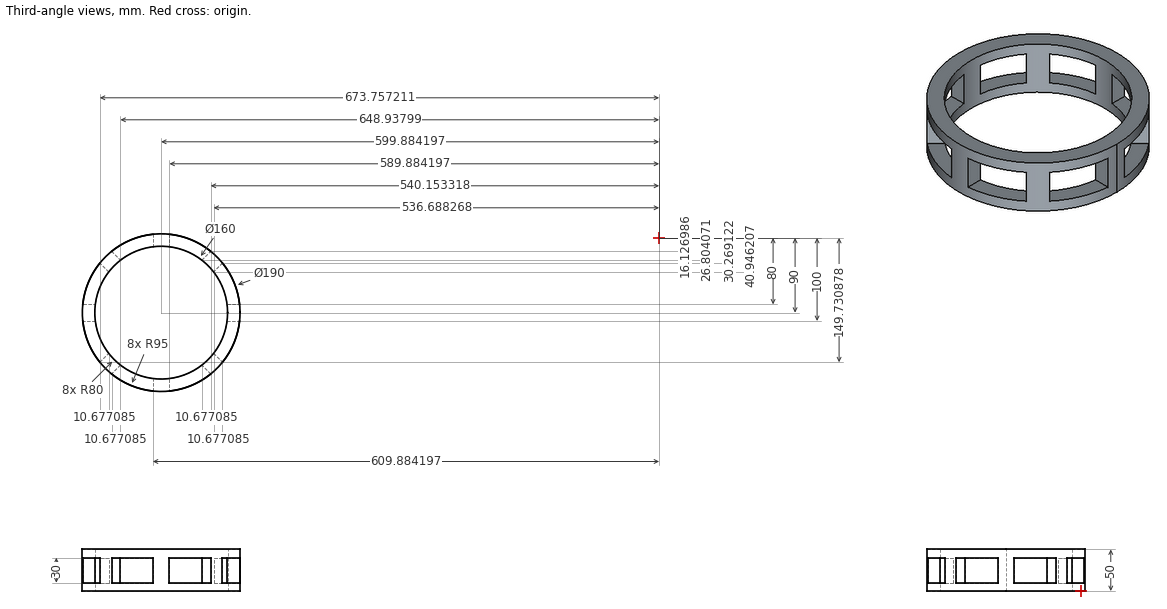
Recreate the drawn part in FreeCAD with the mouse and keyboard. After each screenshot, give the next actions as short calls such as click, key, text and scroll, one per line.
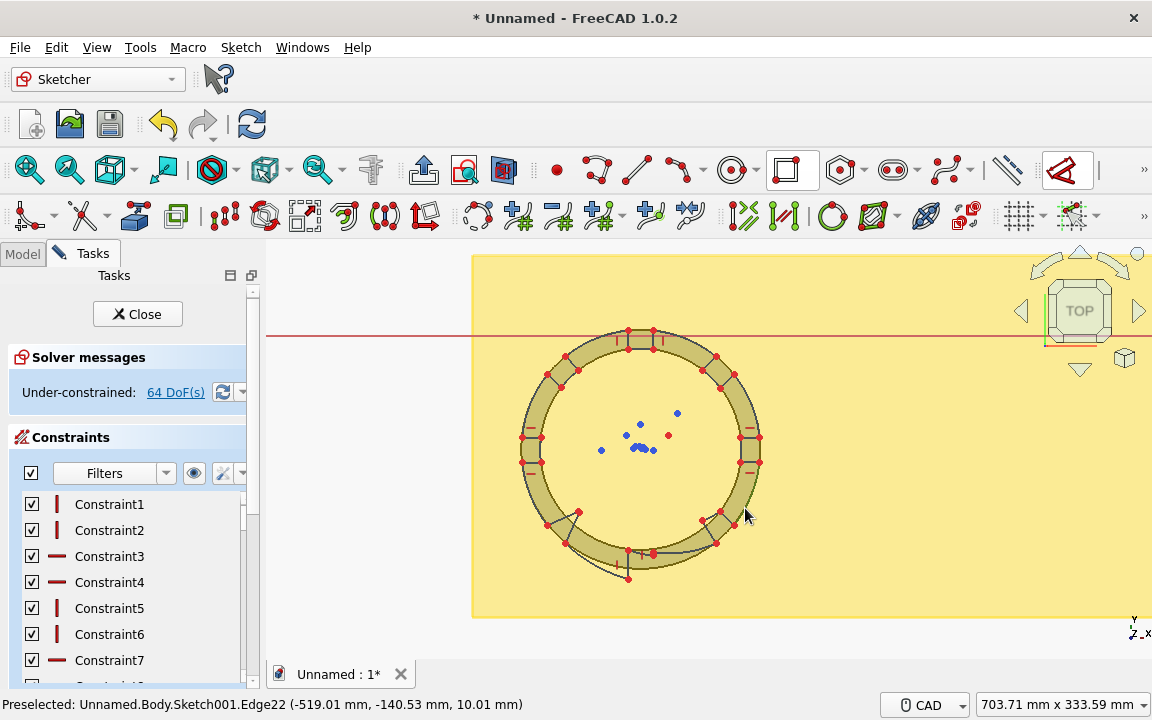
key(c)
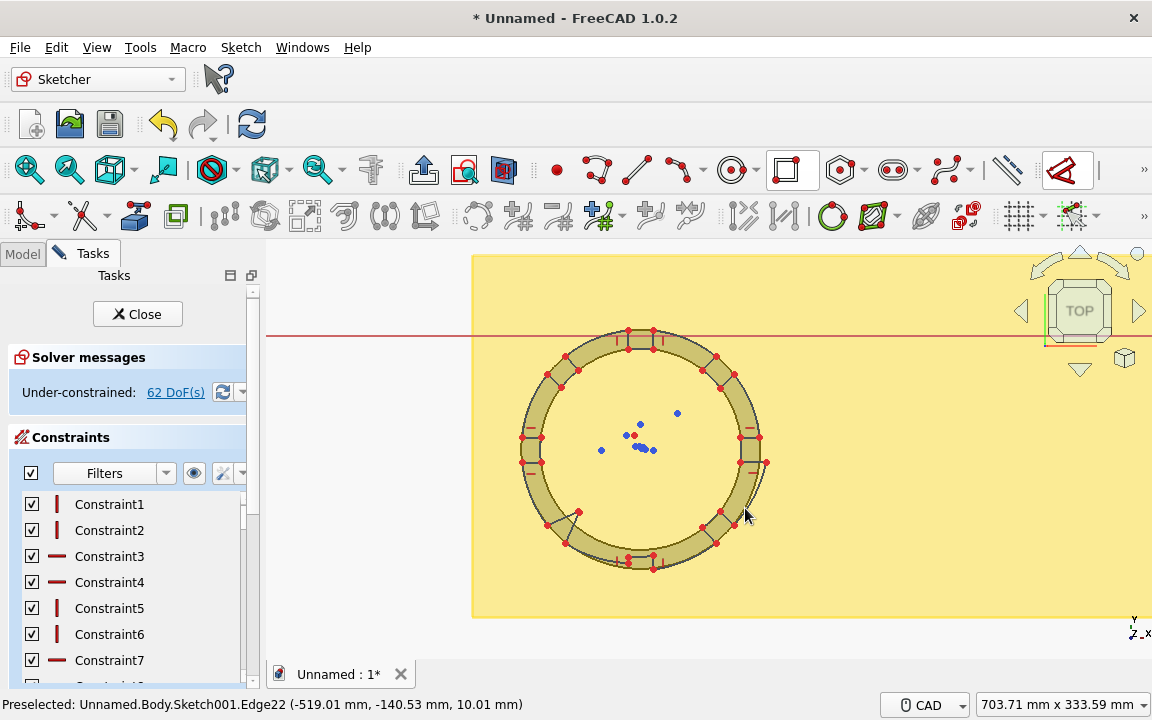
scroll(579, 512, up, 15)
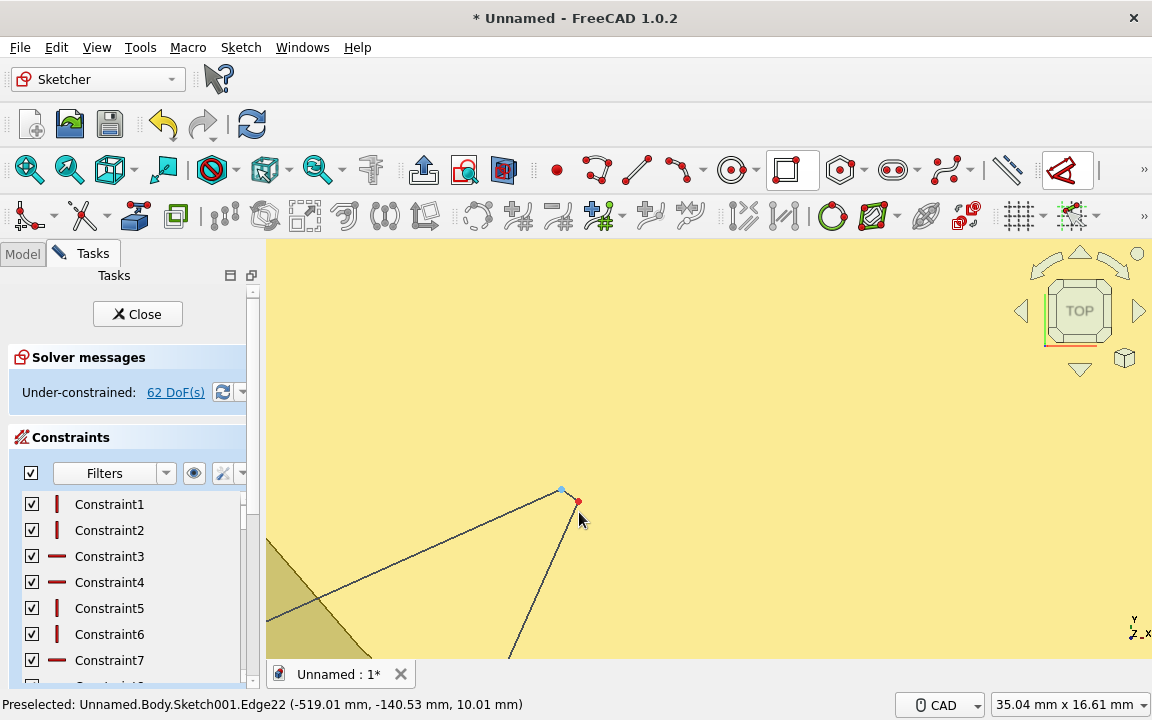
click(570, 495)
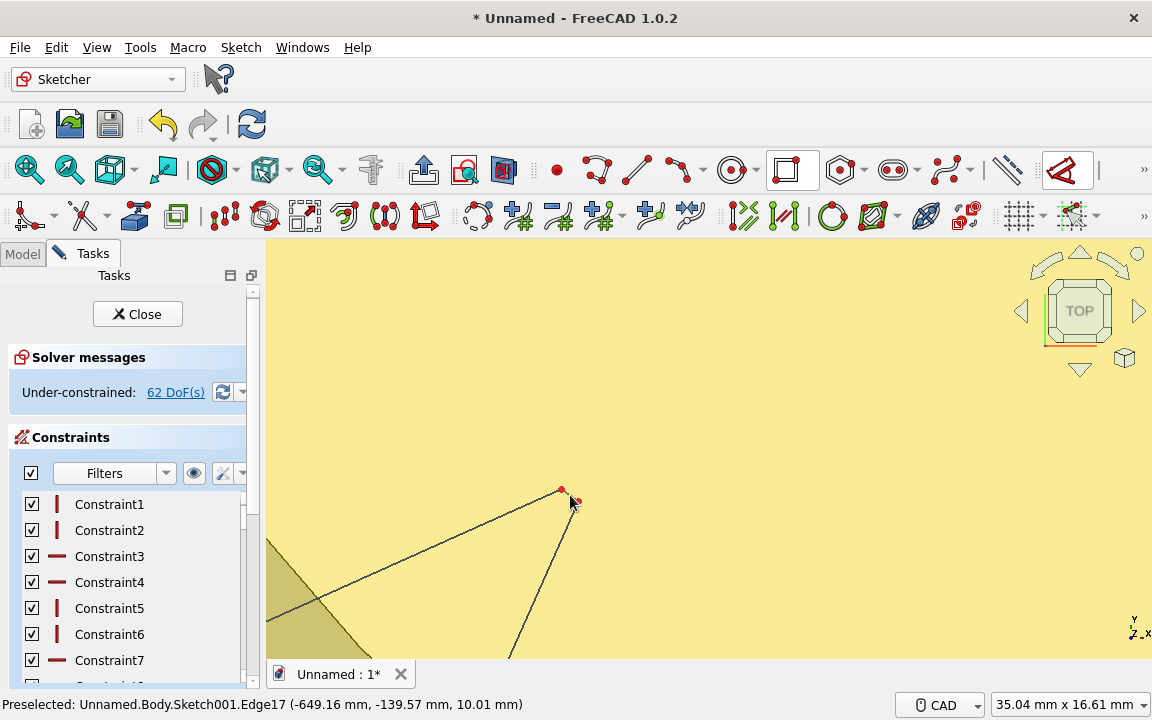
scroll(579, 512, down, 15)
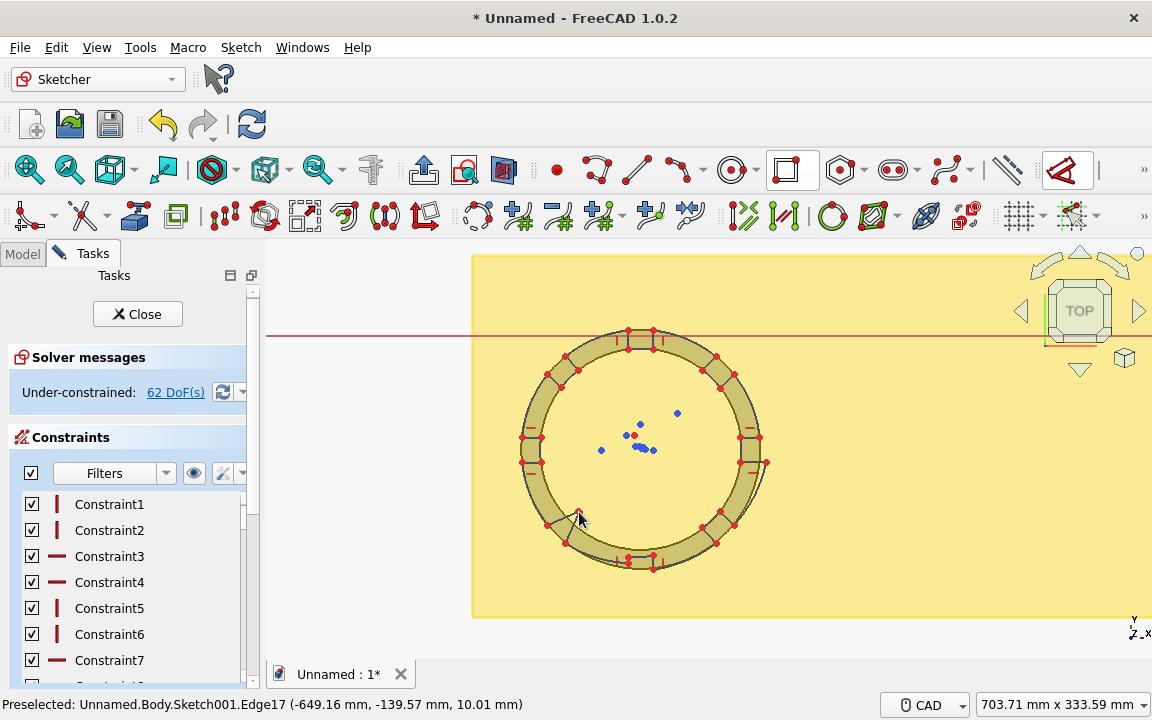
scroll(741, 455, up, 4)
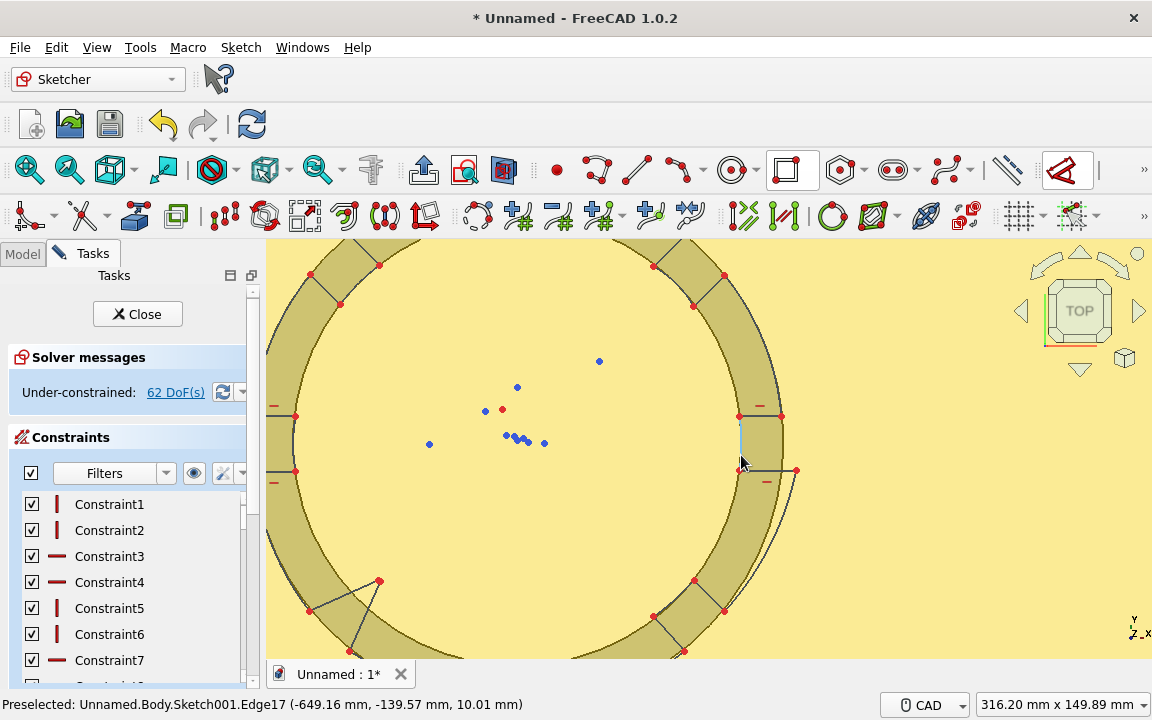
click(741, 454)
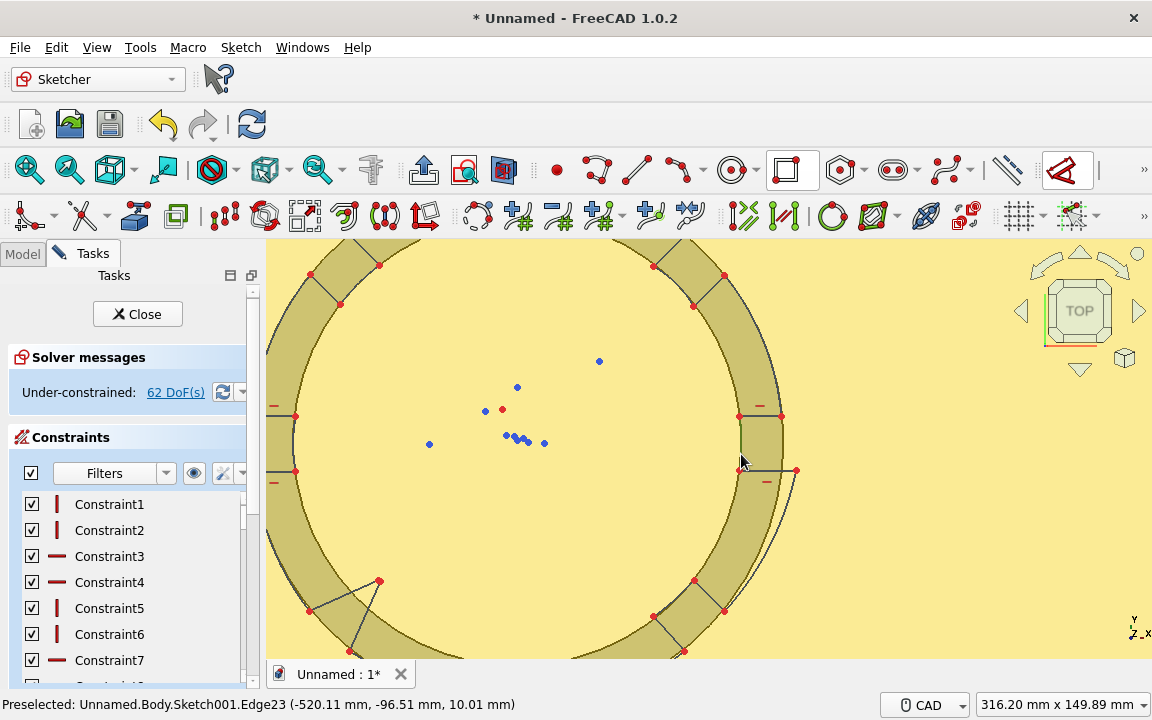
key(c)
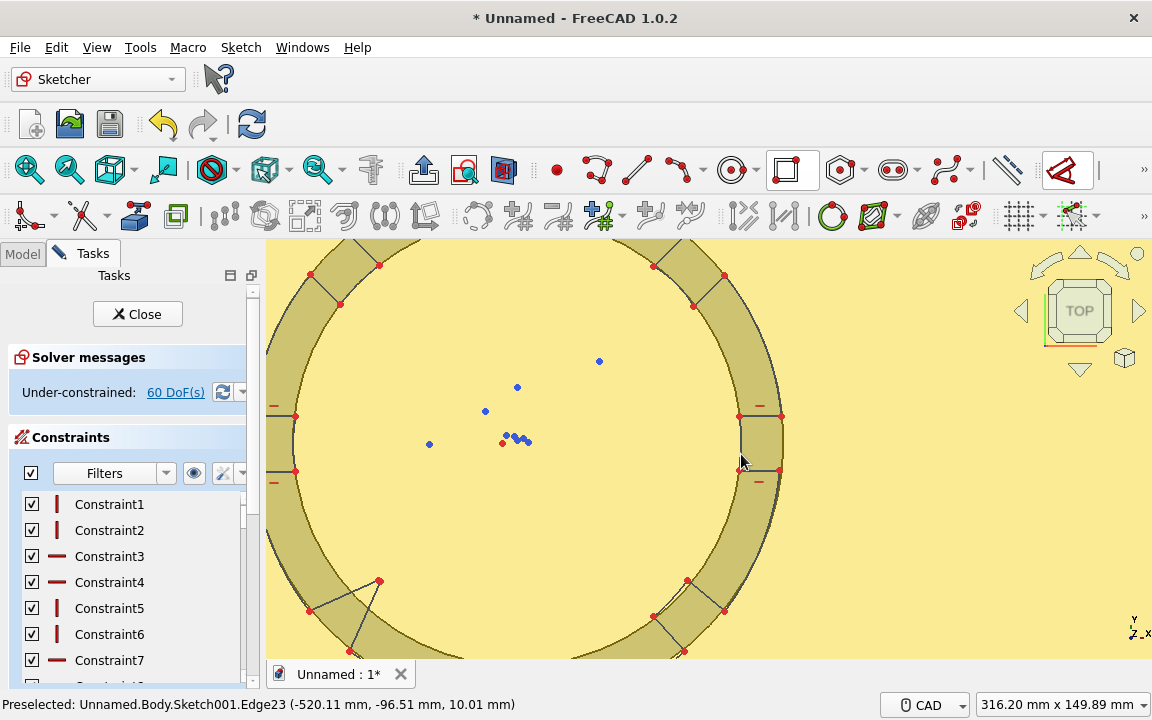
scroll(380, 581, up, 11)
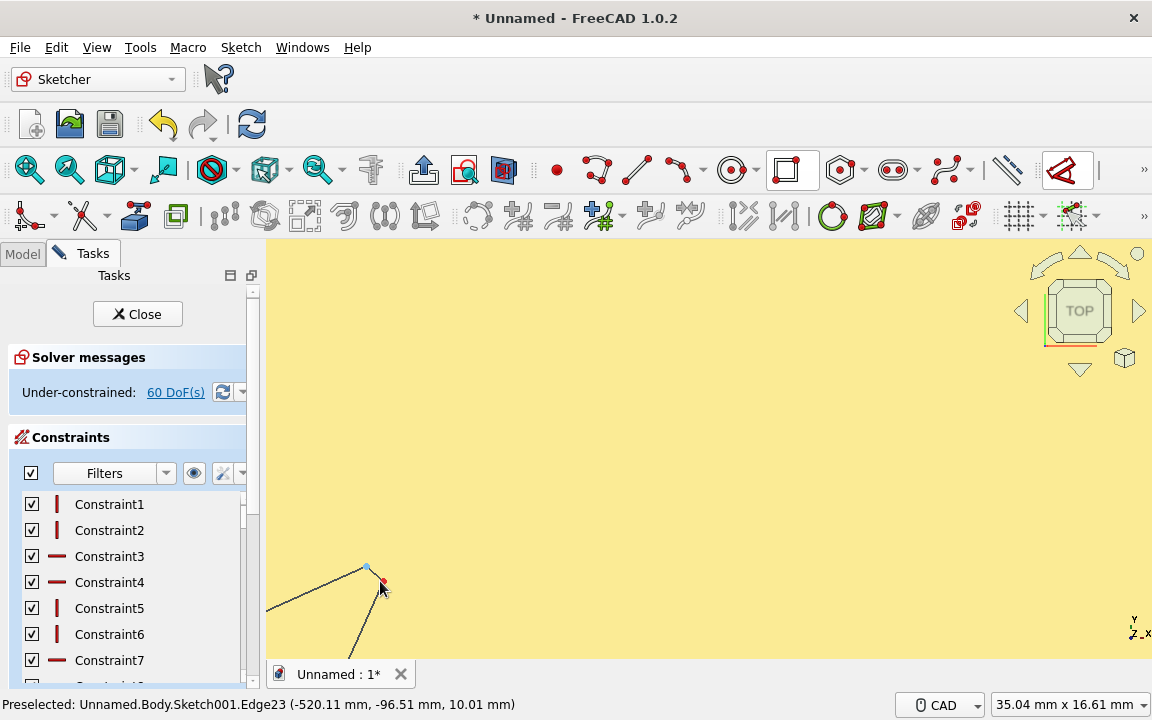
click(375, 574)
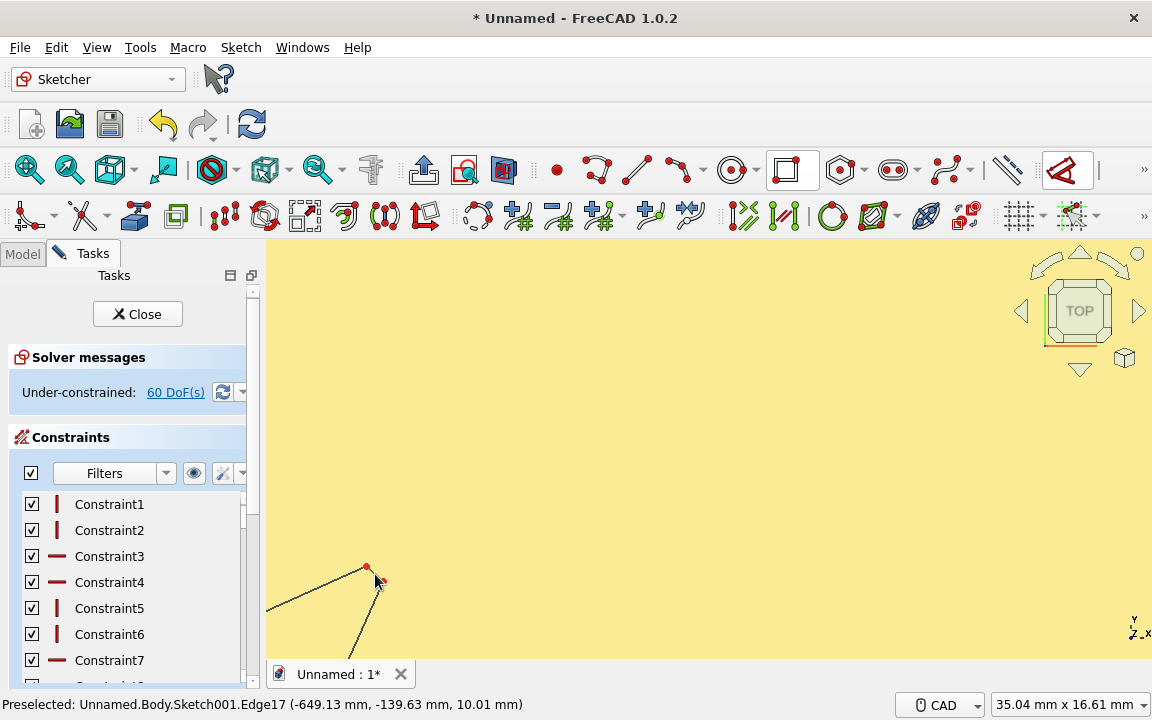
scroll(589, 508, down, 15)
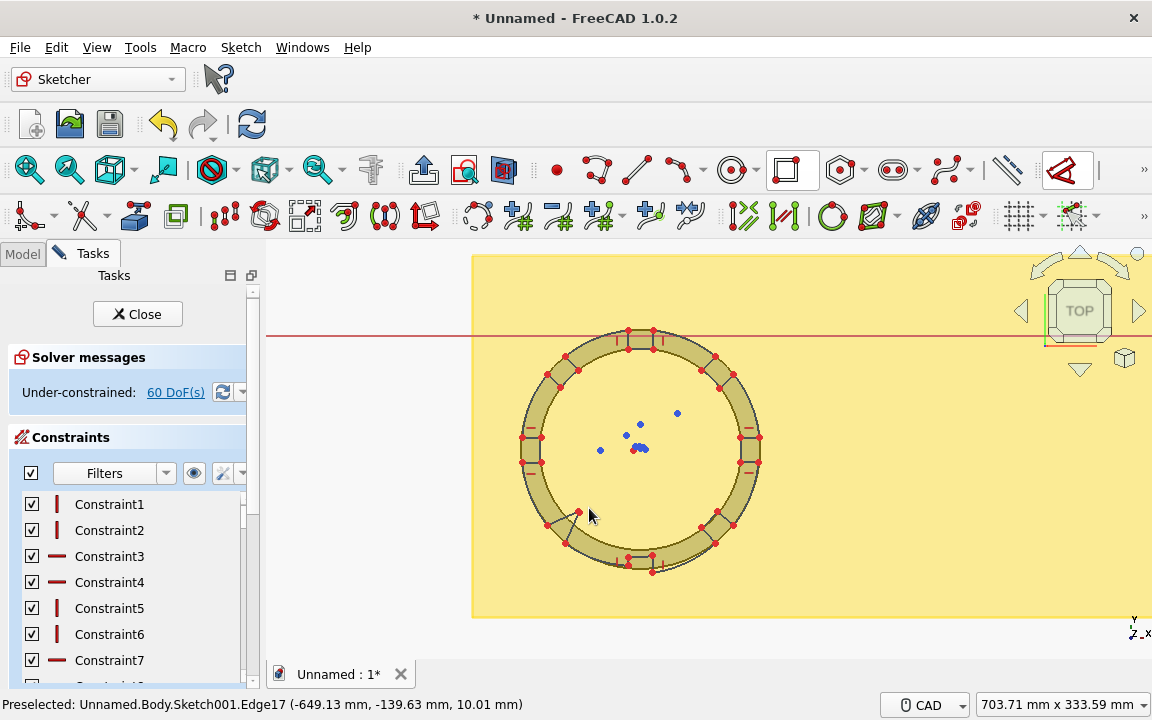
click(756, 417)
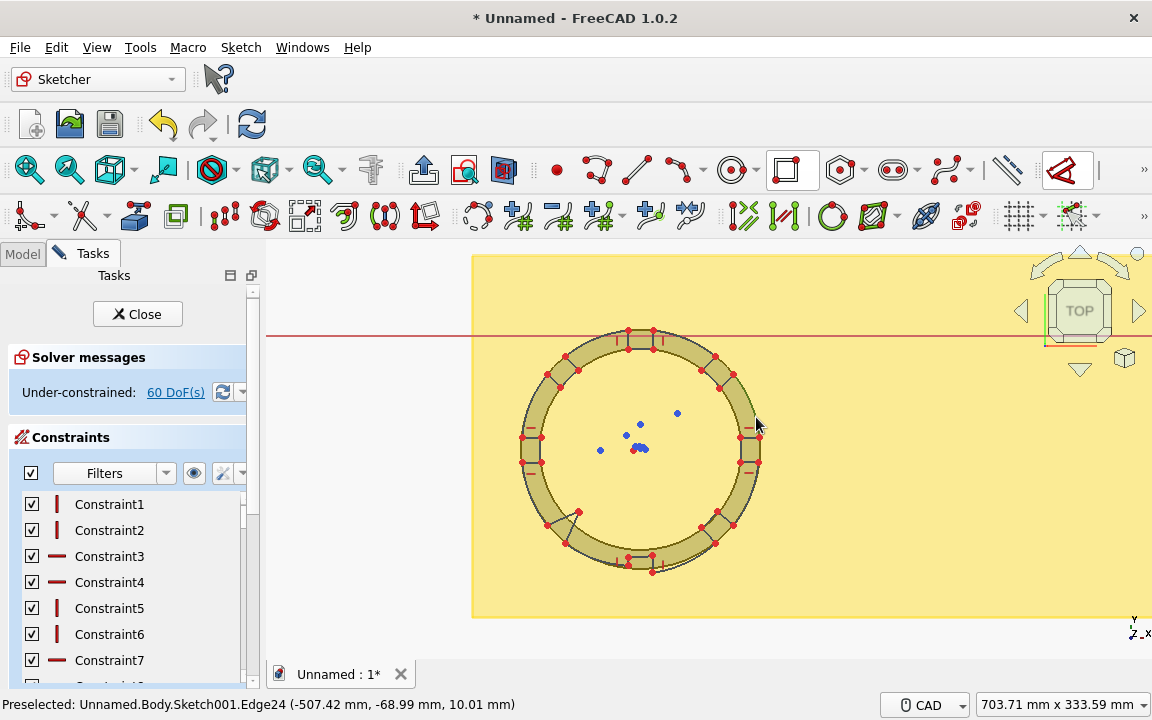
key(c)